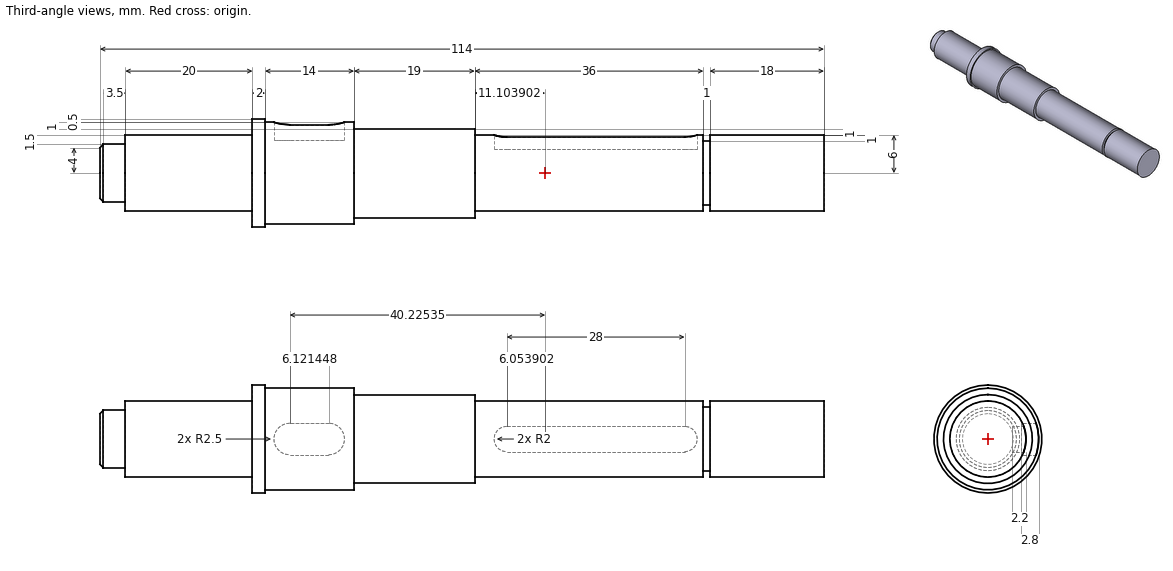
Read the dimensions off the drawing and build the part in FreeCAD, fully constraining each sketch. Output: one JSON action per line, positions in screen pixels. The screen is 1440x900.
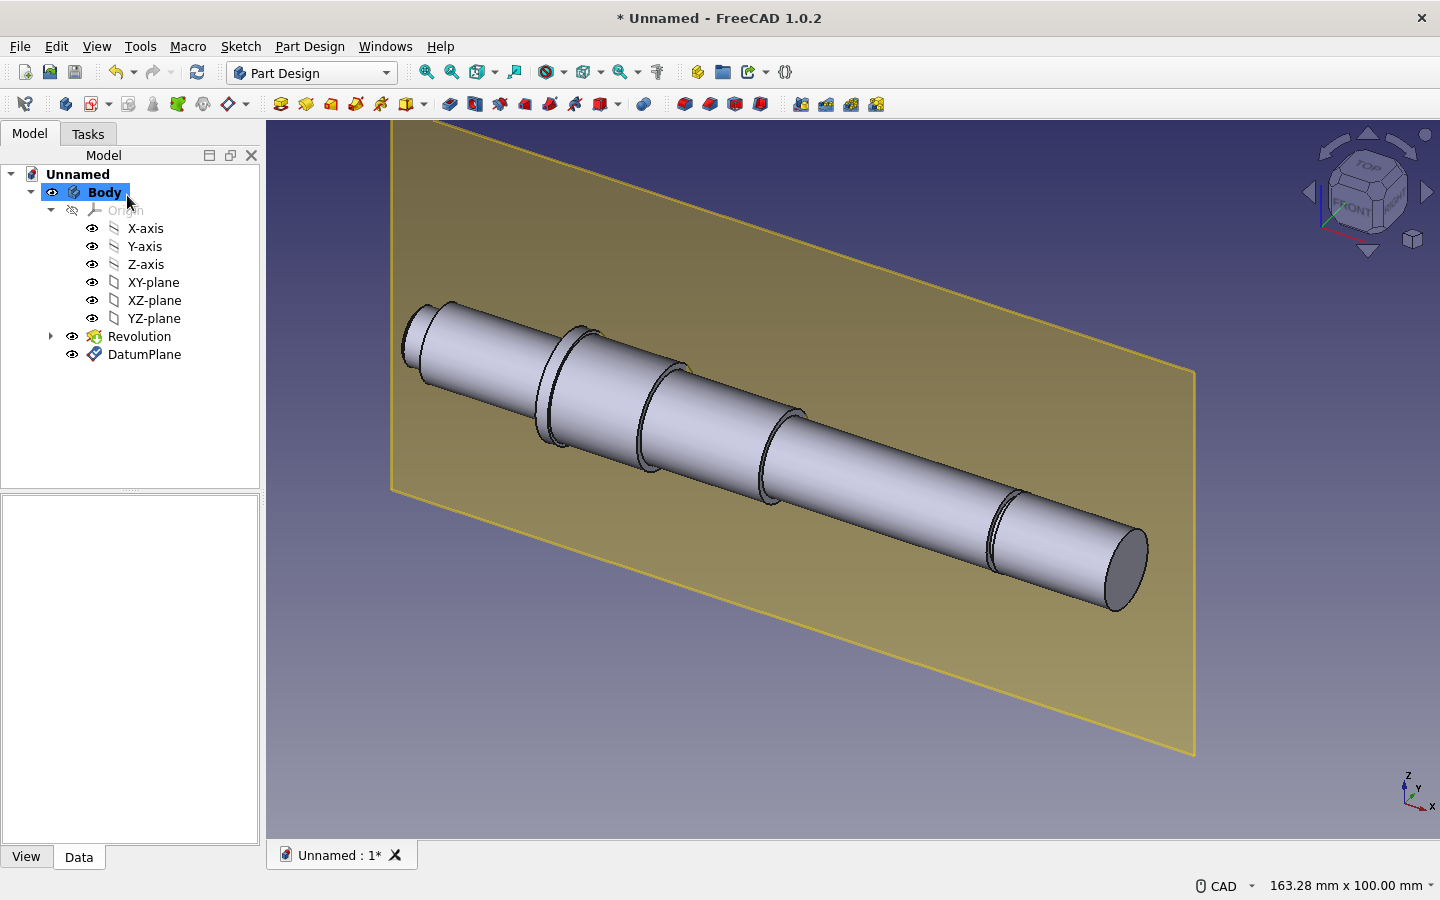
{"action": "left_click", "coordinate": [117, 354]}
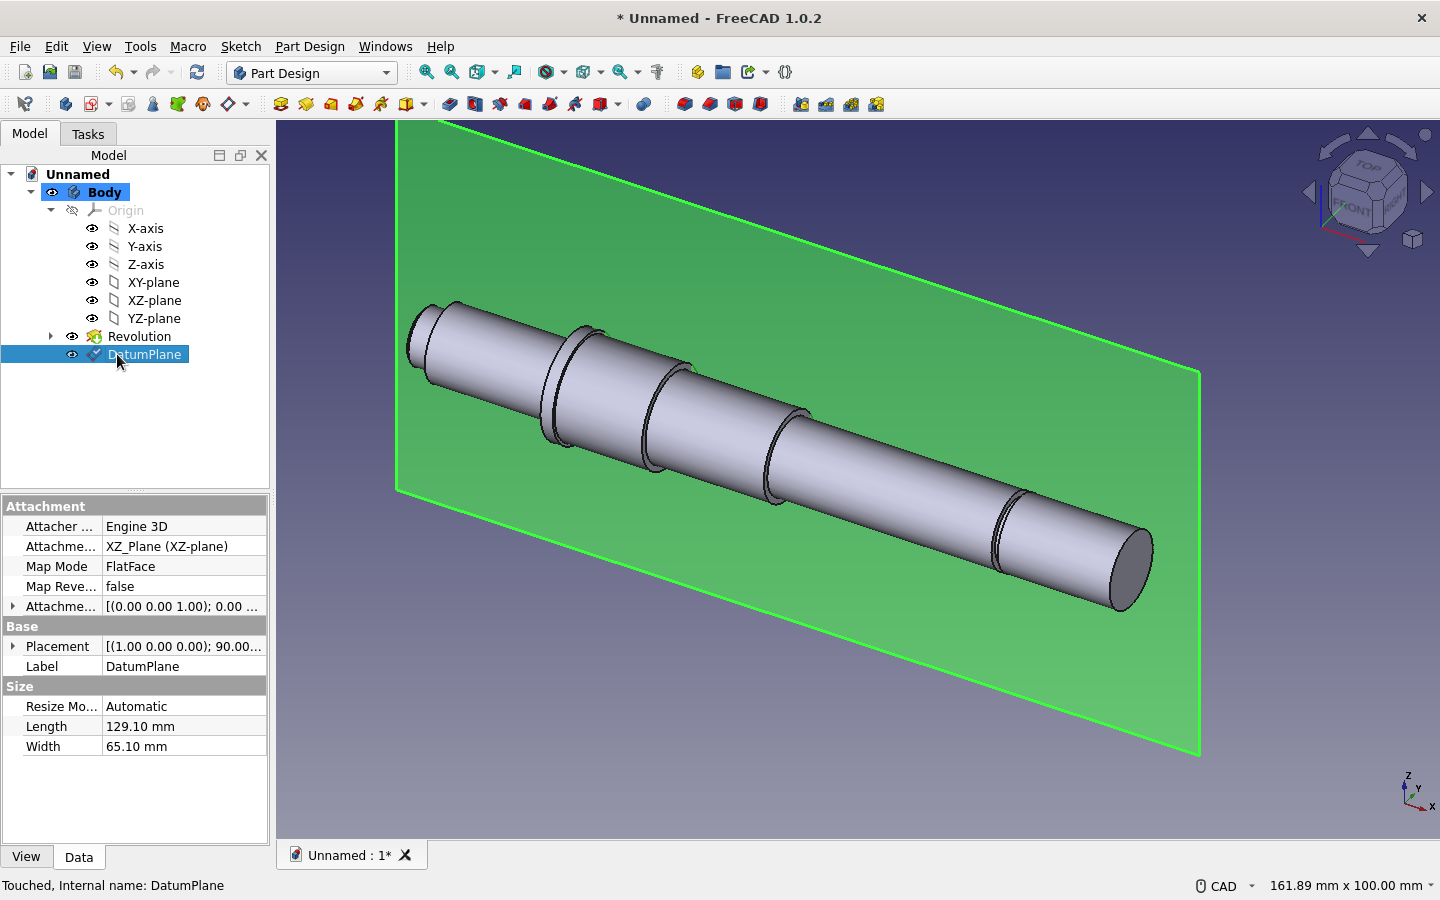
{"action": "left_click", "coordinate": [90, 104]}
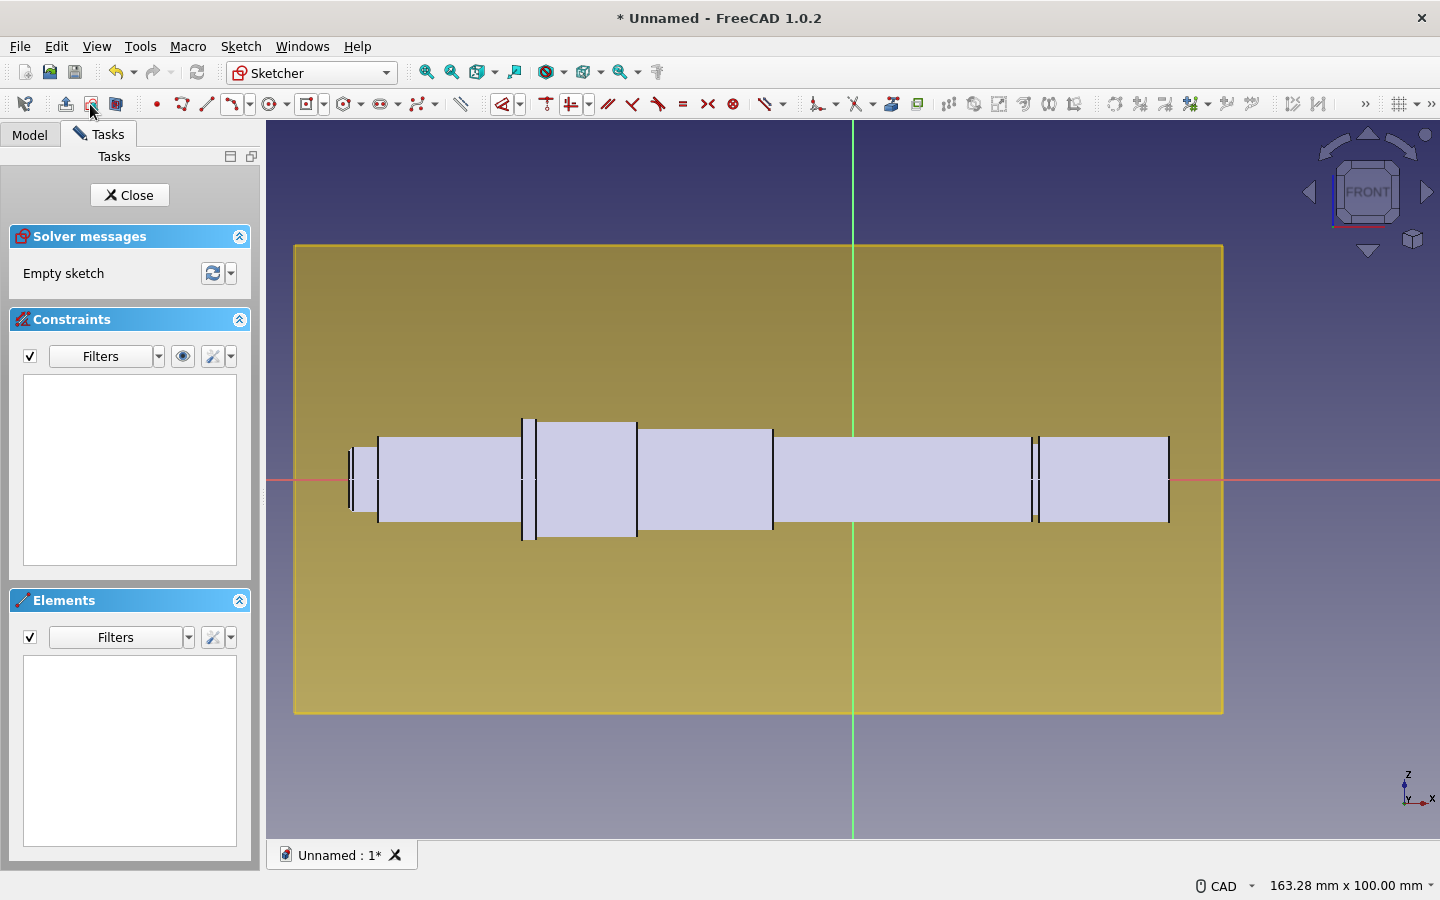
{"action": "left_click", "coordinate": [116, 104]}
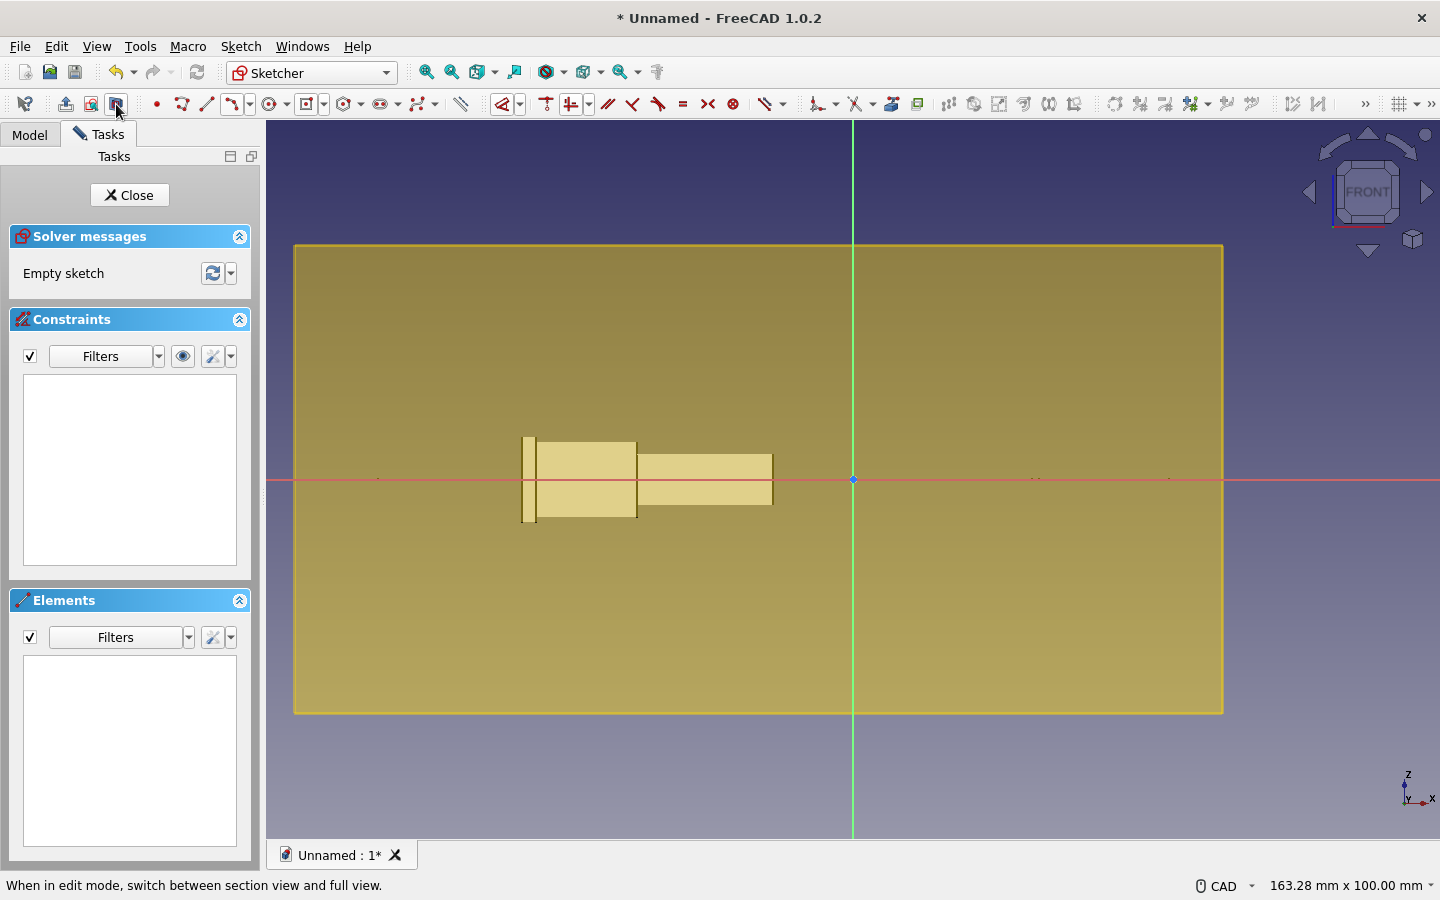
{"action": "scroll", "coordinate": [964, 480], "scroll_direction": "up", "scroll_amount": 6}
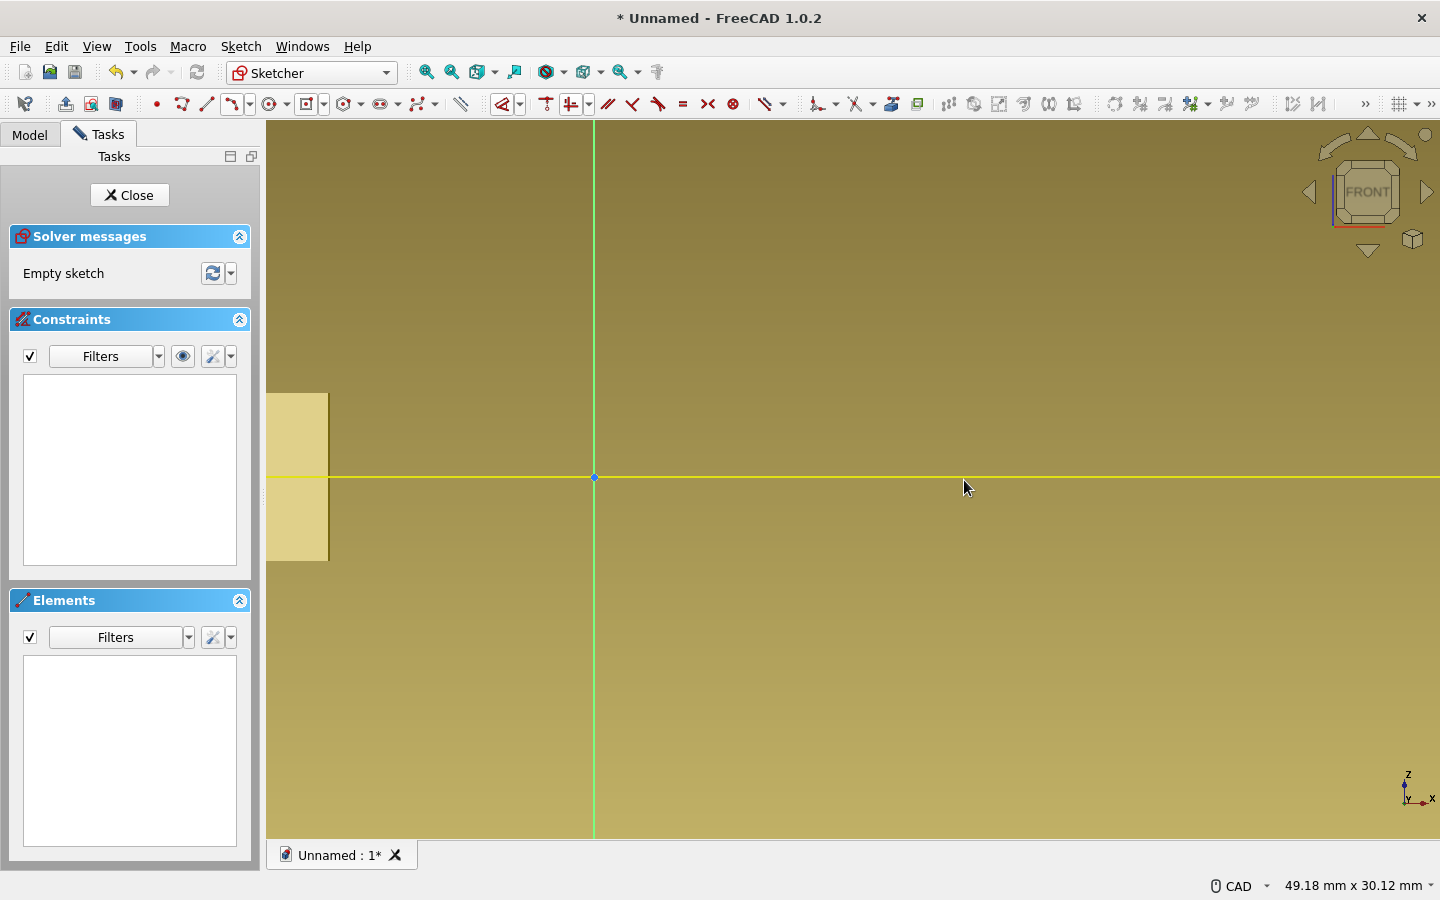
{"action": "left_click", "coordinate": [380, 104]}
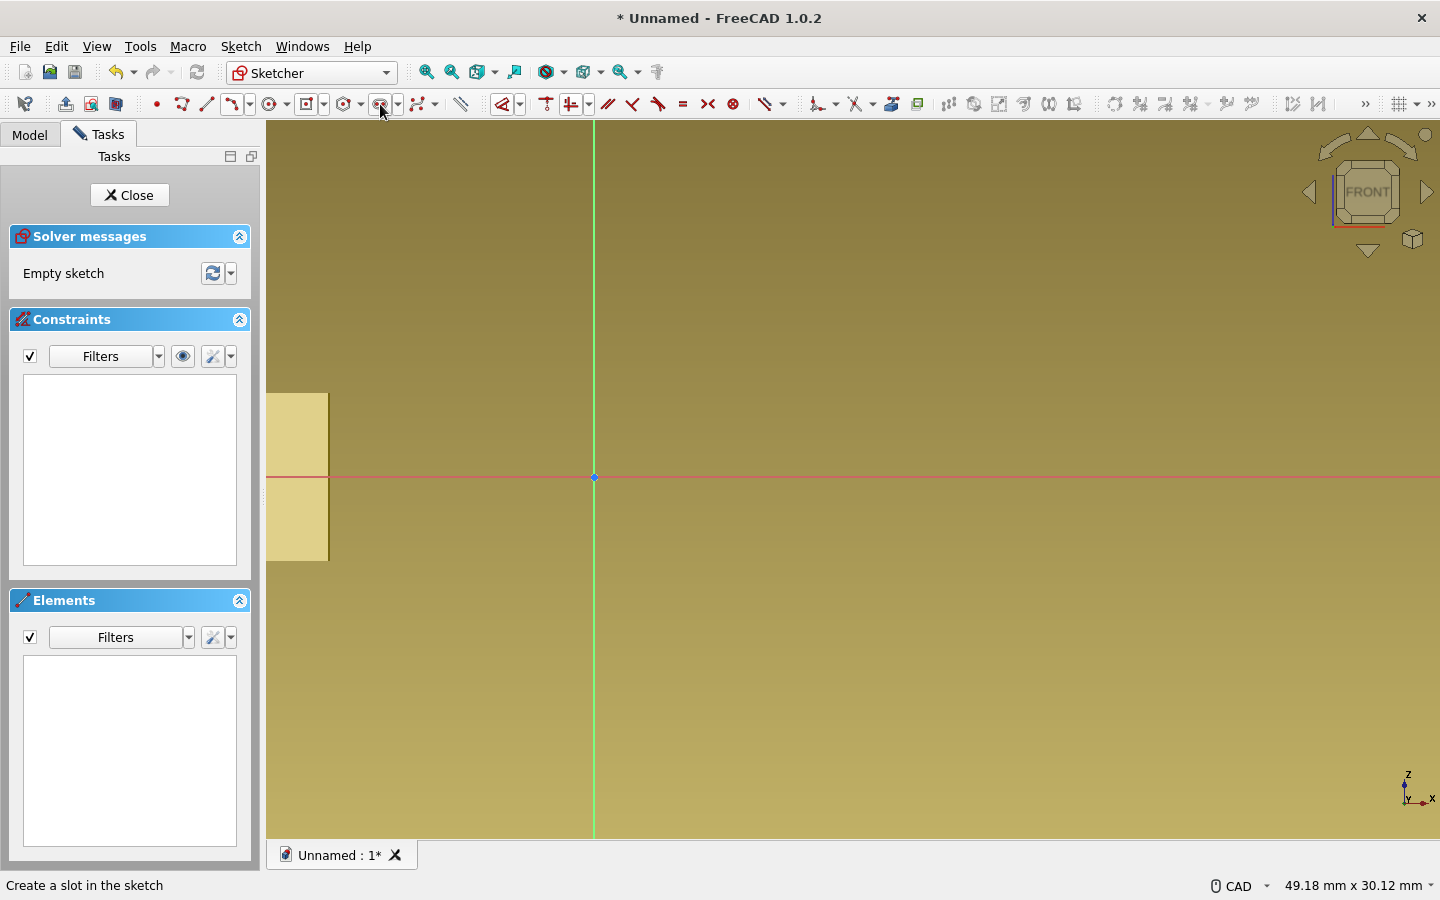
{"action": "left_click", "coordinate": [450, 477]}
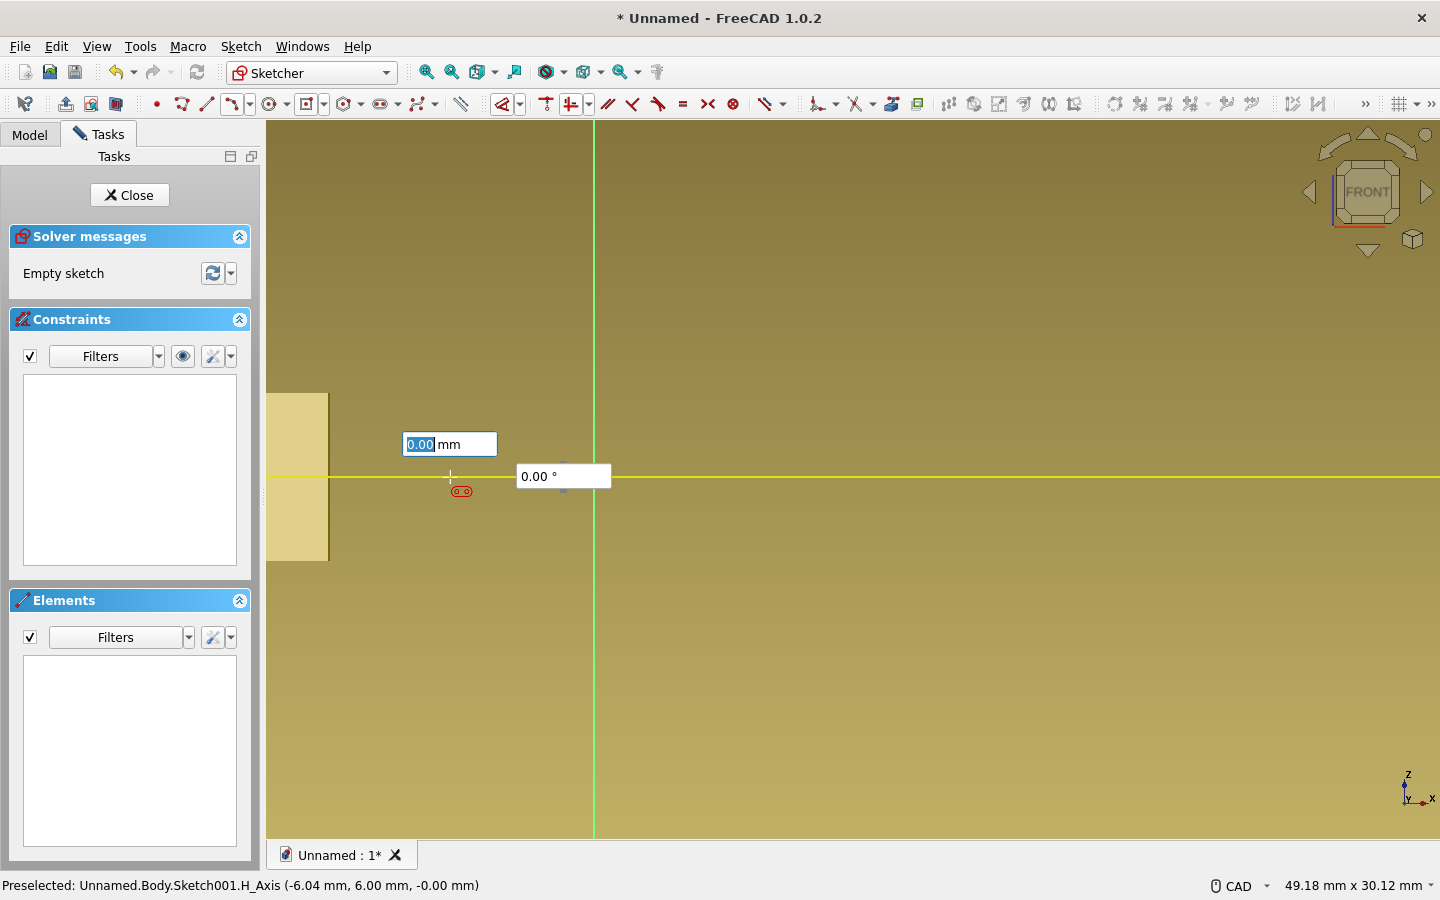
{"action": "left_click", "coordinate": [1118, 468]}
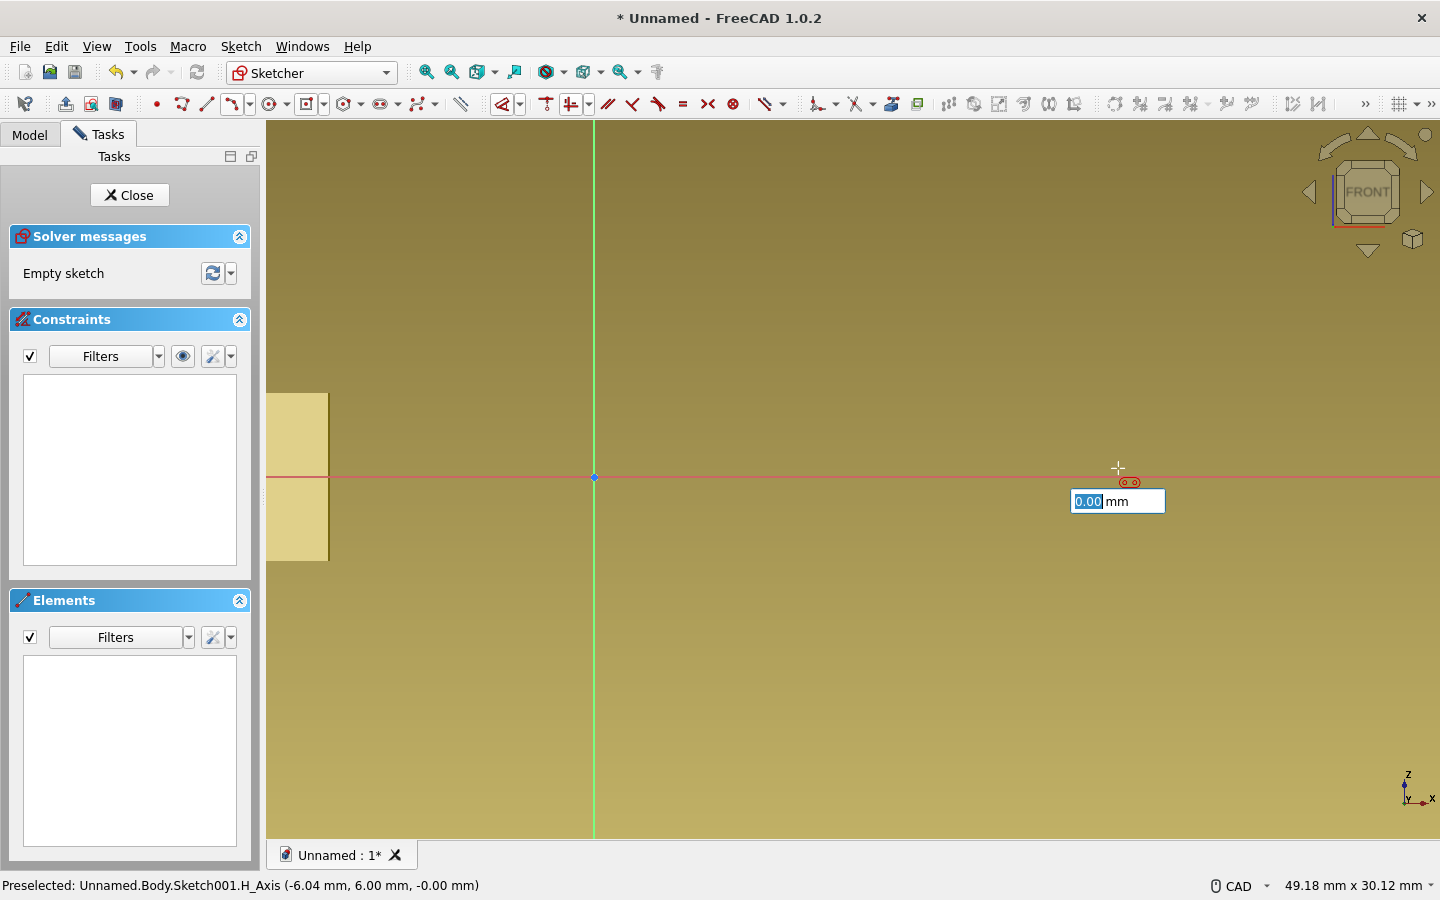
{"action": "left_click", "coordinate": [784, 525]}
{"action": "key", "text": "Escape"}